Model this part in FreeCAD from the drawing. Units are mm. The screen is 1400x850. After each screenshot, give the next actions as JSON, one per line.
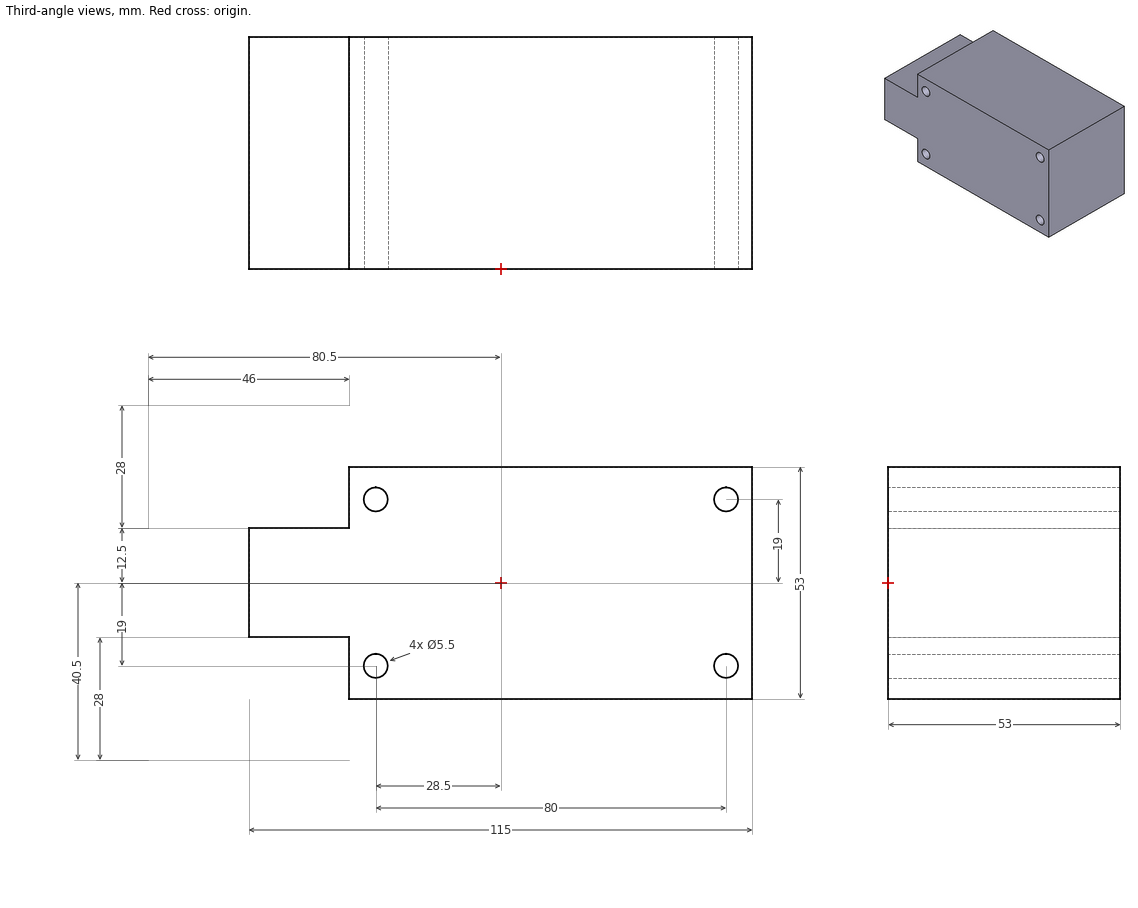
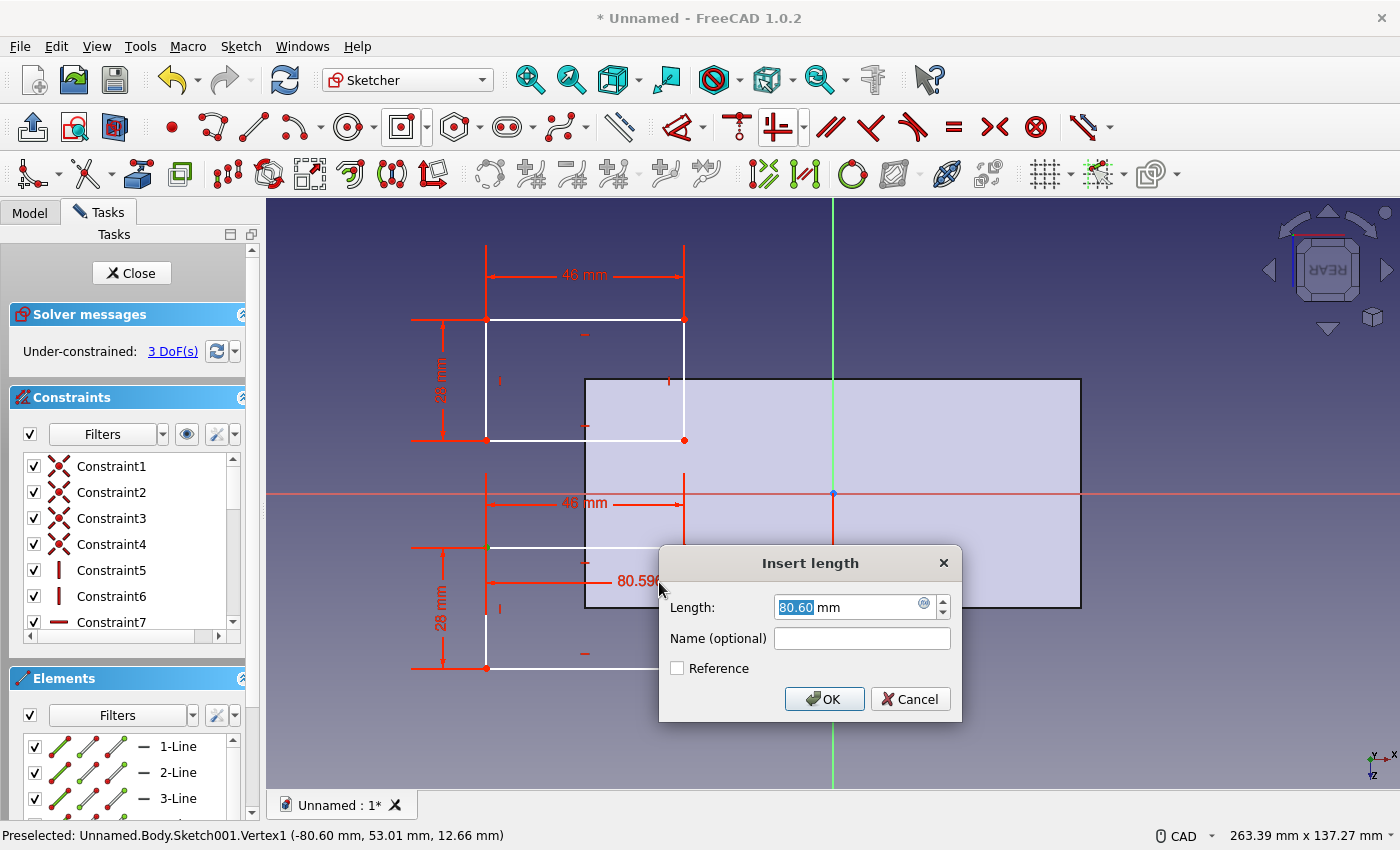
{"action": "type", "text": "80.5"}
{"action": "key", "text": "Return"}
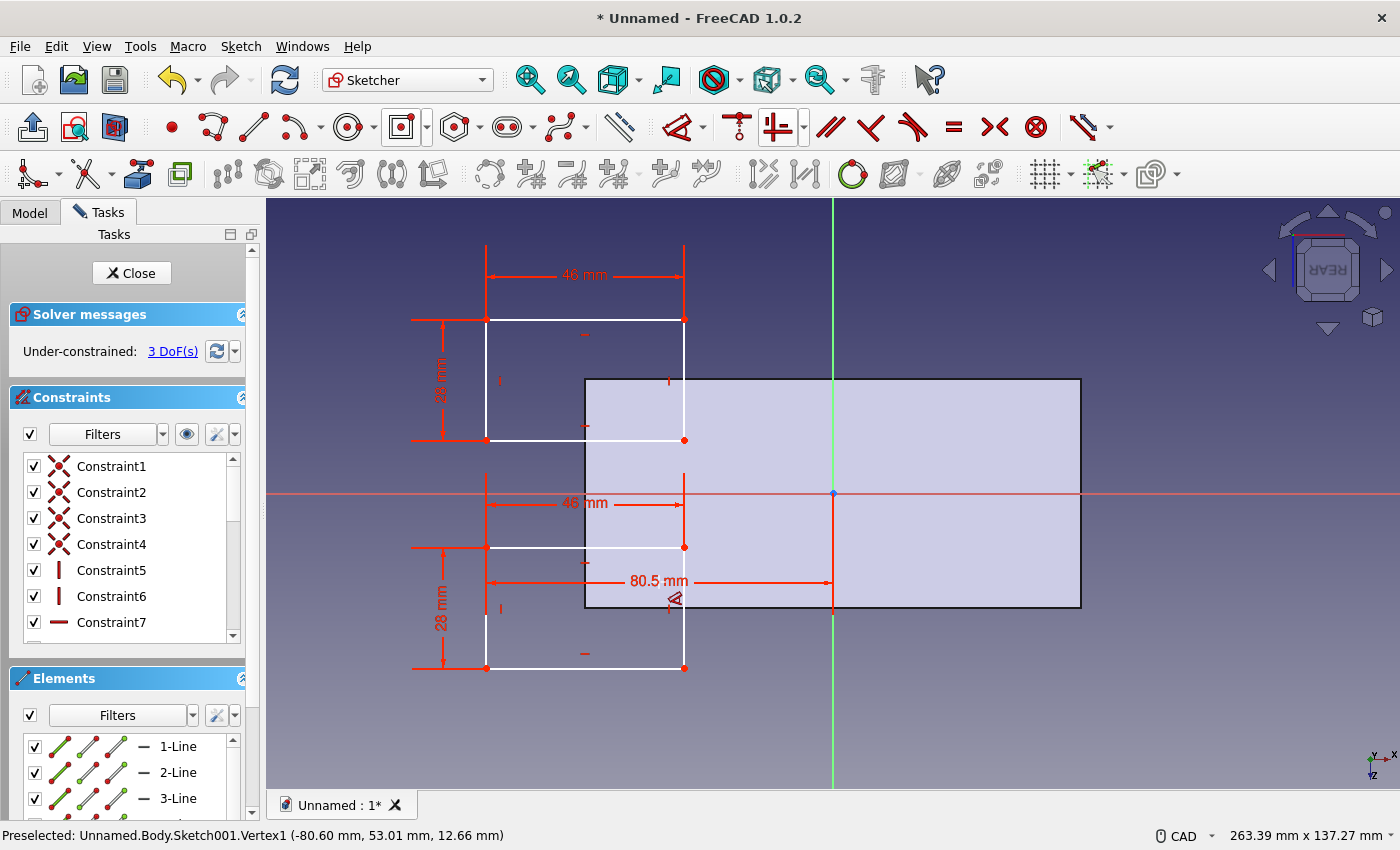
{"action": "left_click", "coordinate": [486, 548]}
{"action": "left_click", "coordinate": [867, 521]}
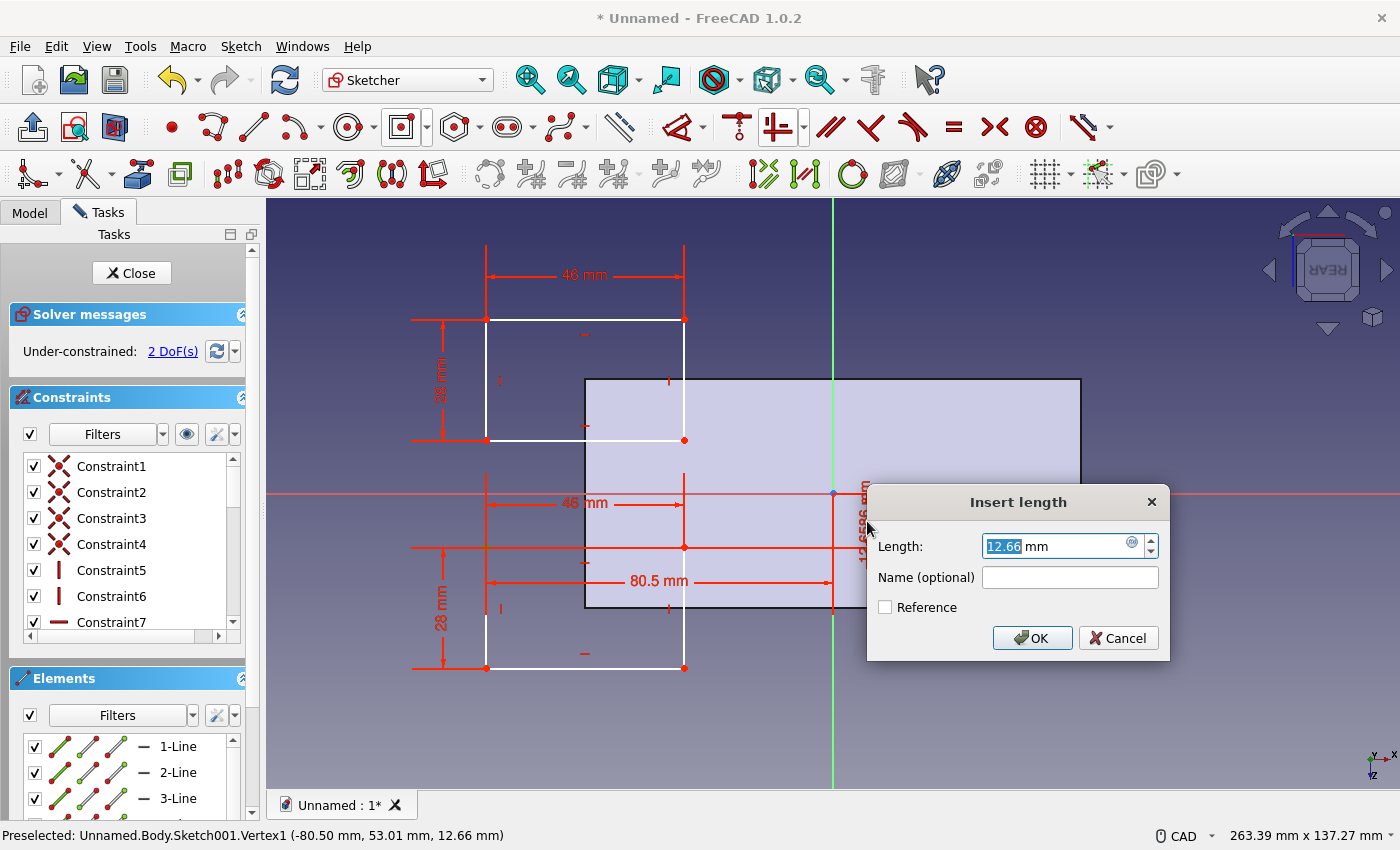
{"action": "type", "text": "12.5"}
{"action": "key", "text": "Return"}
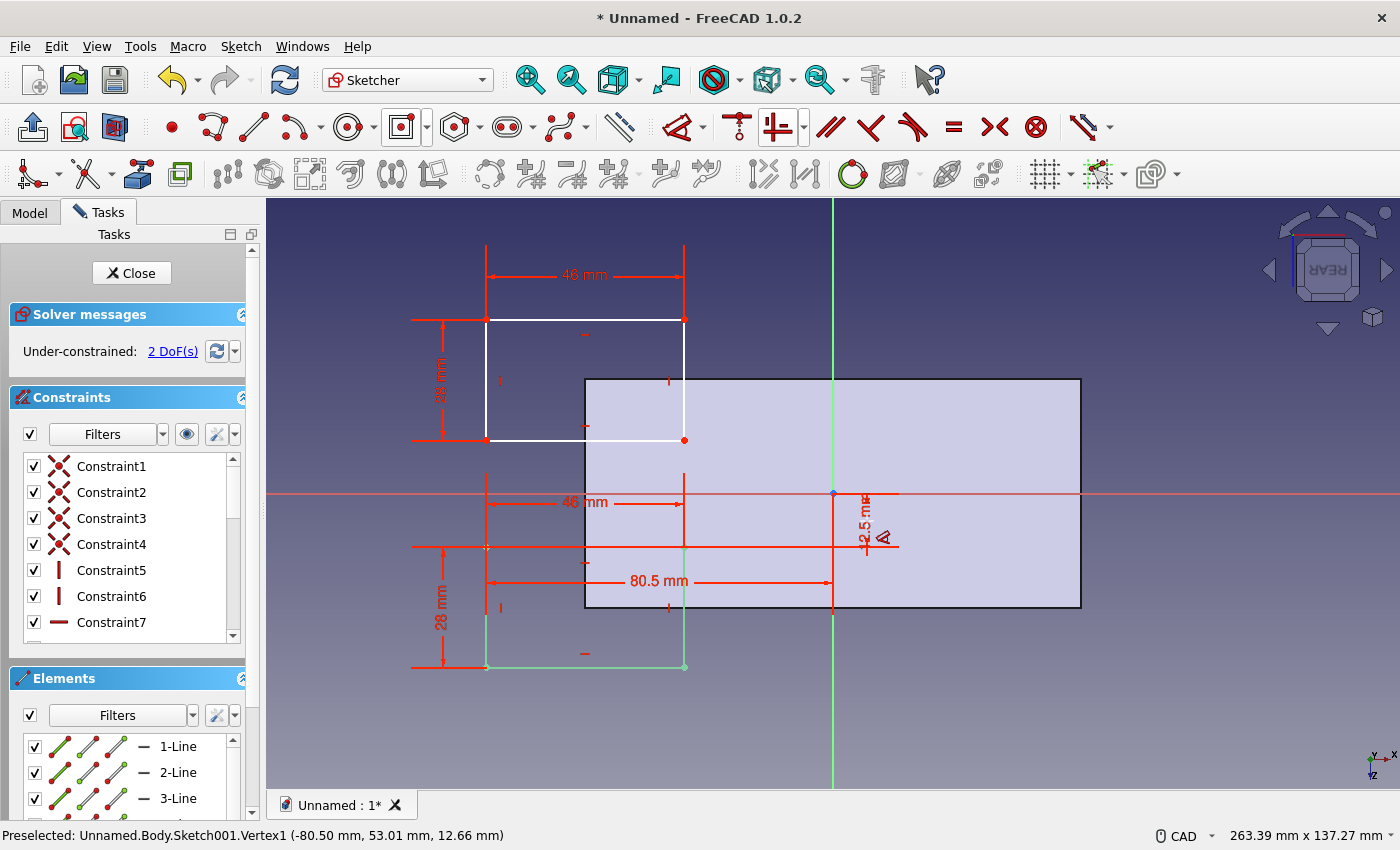
{"action": "left_click", "coordinate": [486, 320]}
{"action": "left_click", "coordinate": [659, 286]}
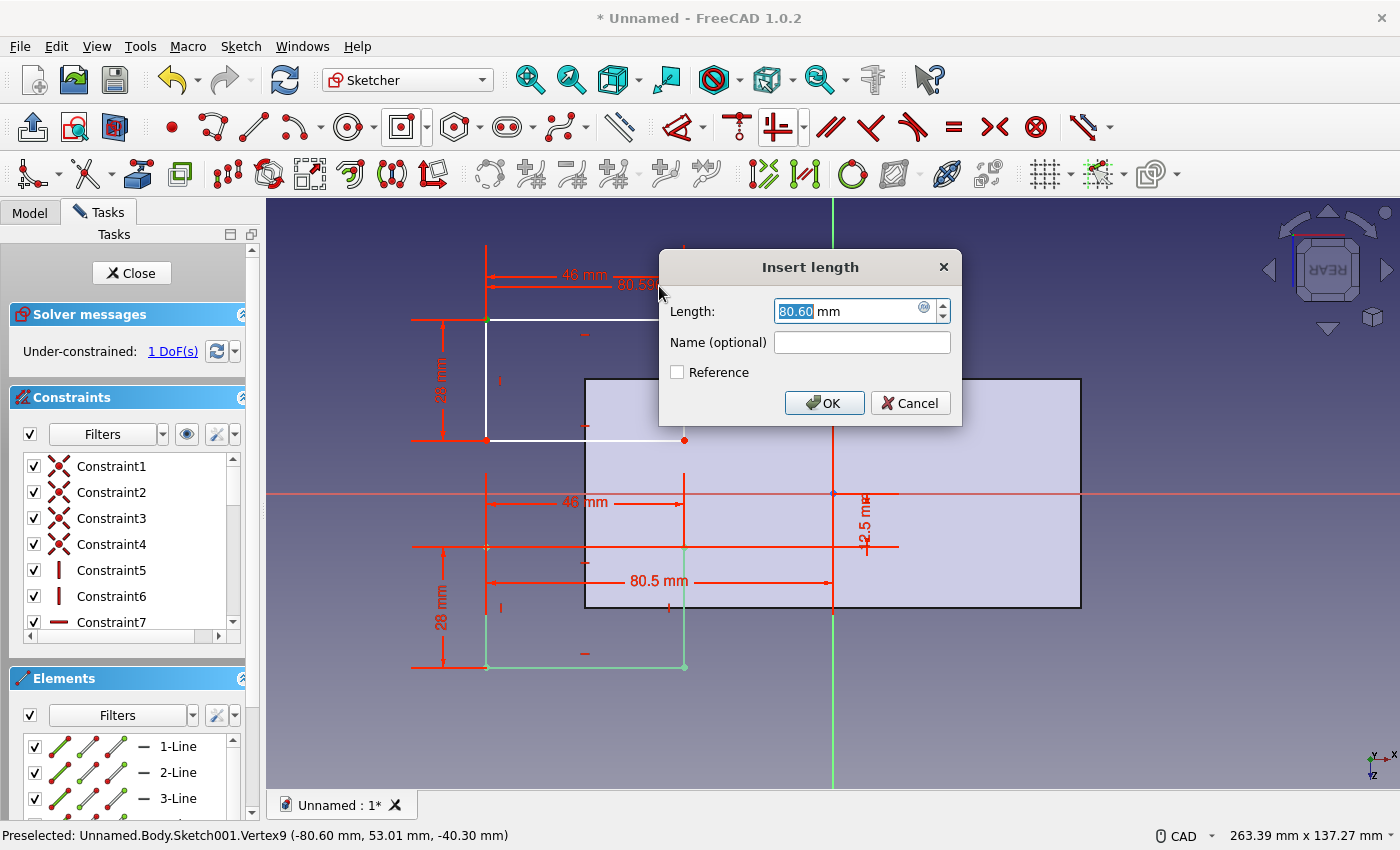
{"action": "type", "text": "80.5"}
{"action": "key", "text": "Return"}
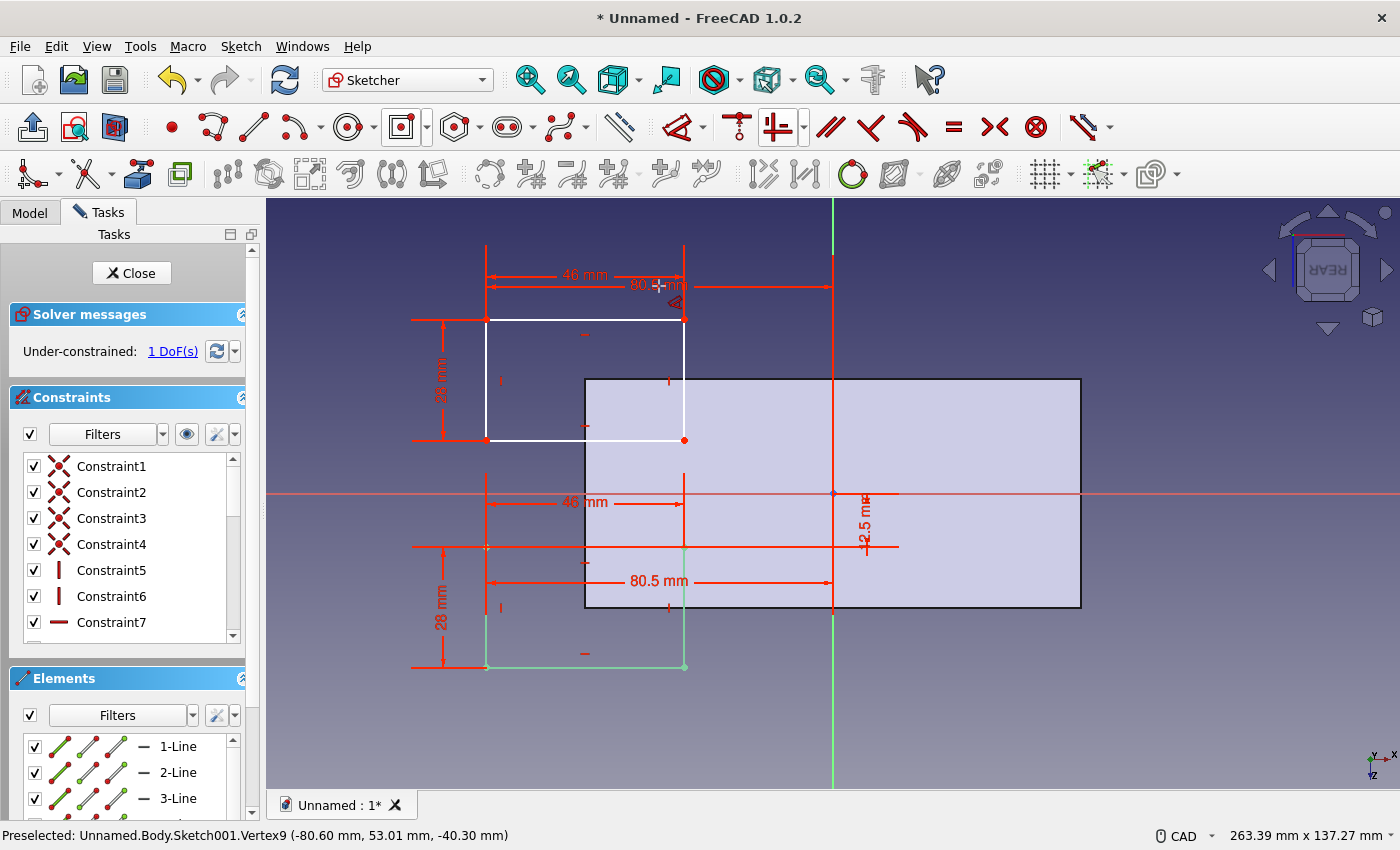
{"action": "left_click", "coordinate": [486, 320]}
{"action": "left_click", "coordinate": [867, 407]}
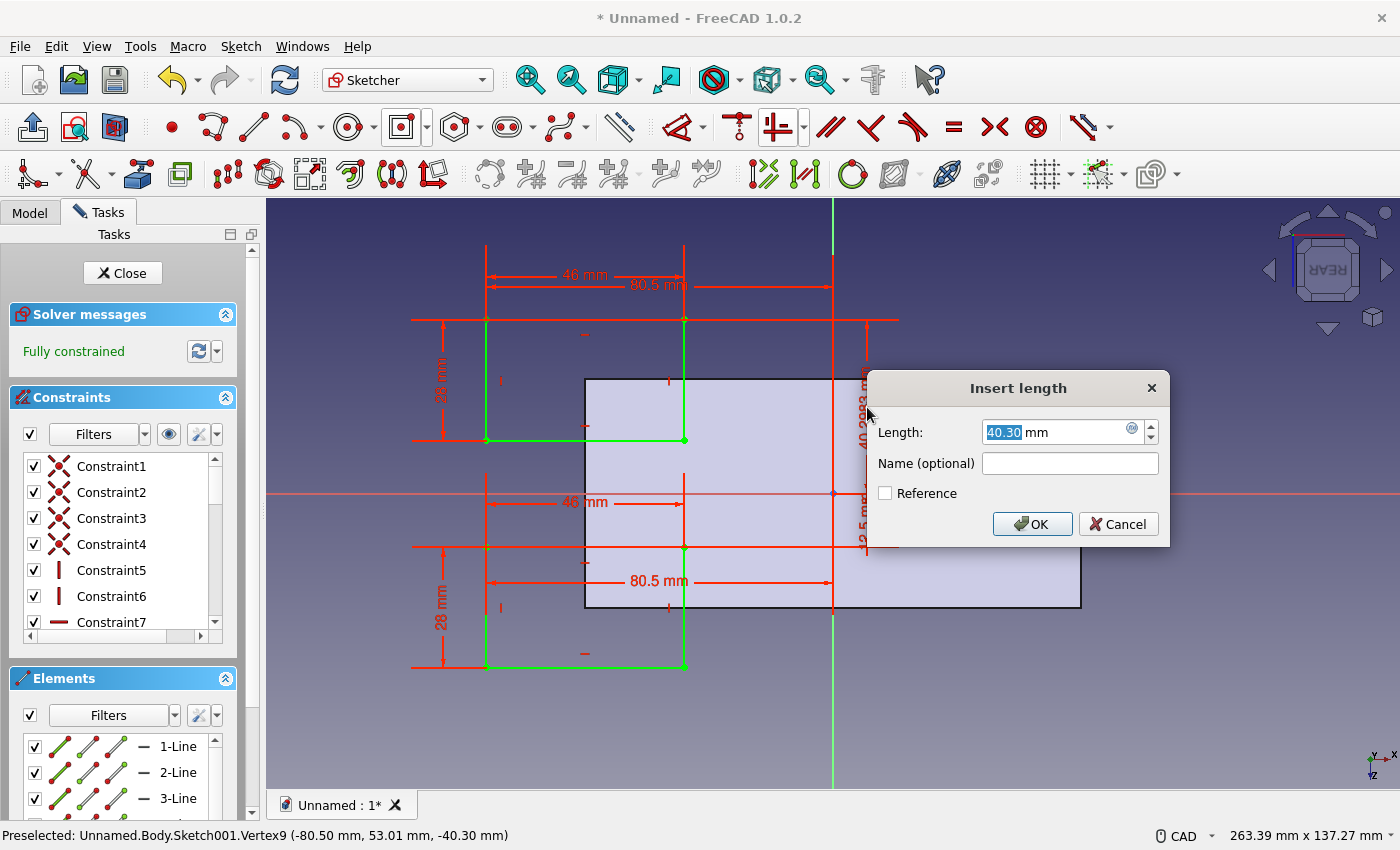
{"action": "type", "text": "40.5"}
{"action": "key", "text": "Return"}
{"action": "key", "text": "Escape"}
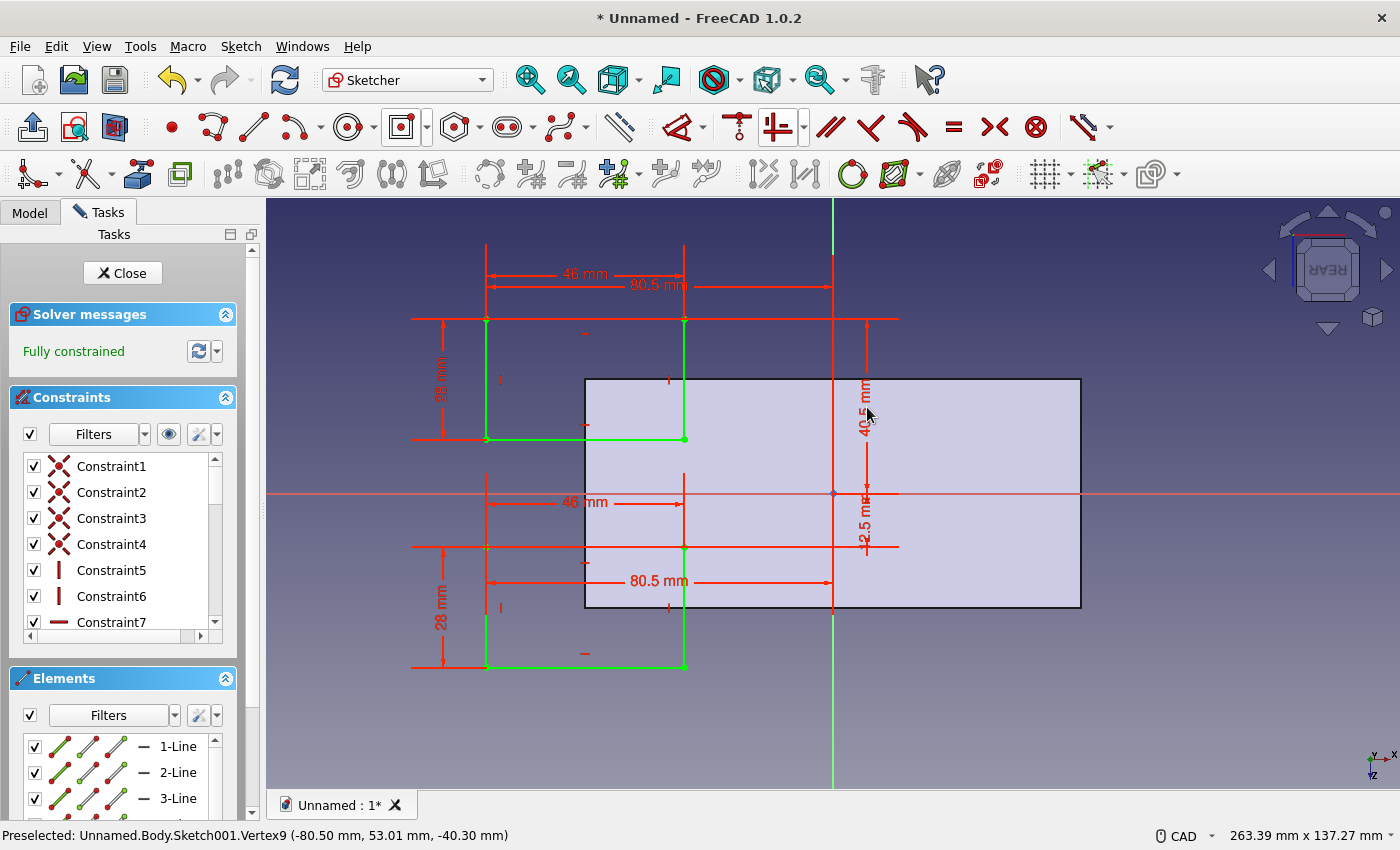
{"action": "left_click", "coordinate": [123, 273]}